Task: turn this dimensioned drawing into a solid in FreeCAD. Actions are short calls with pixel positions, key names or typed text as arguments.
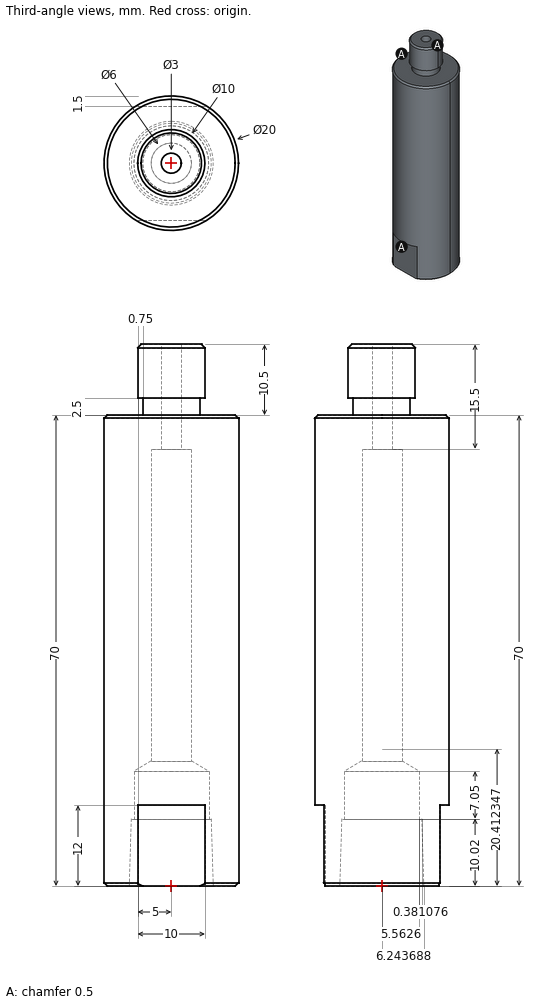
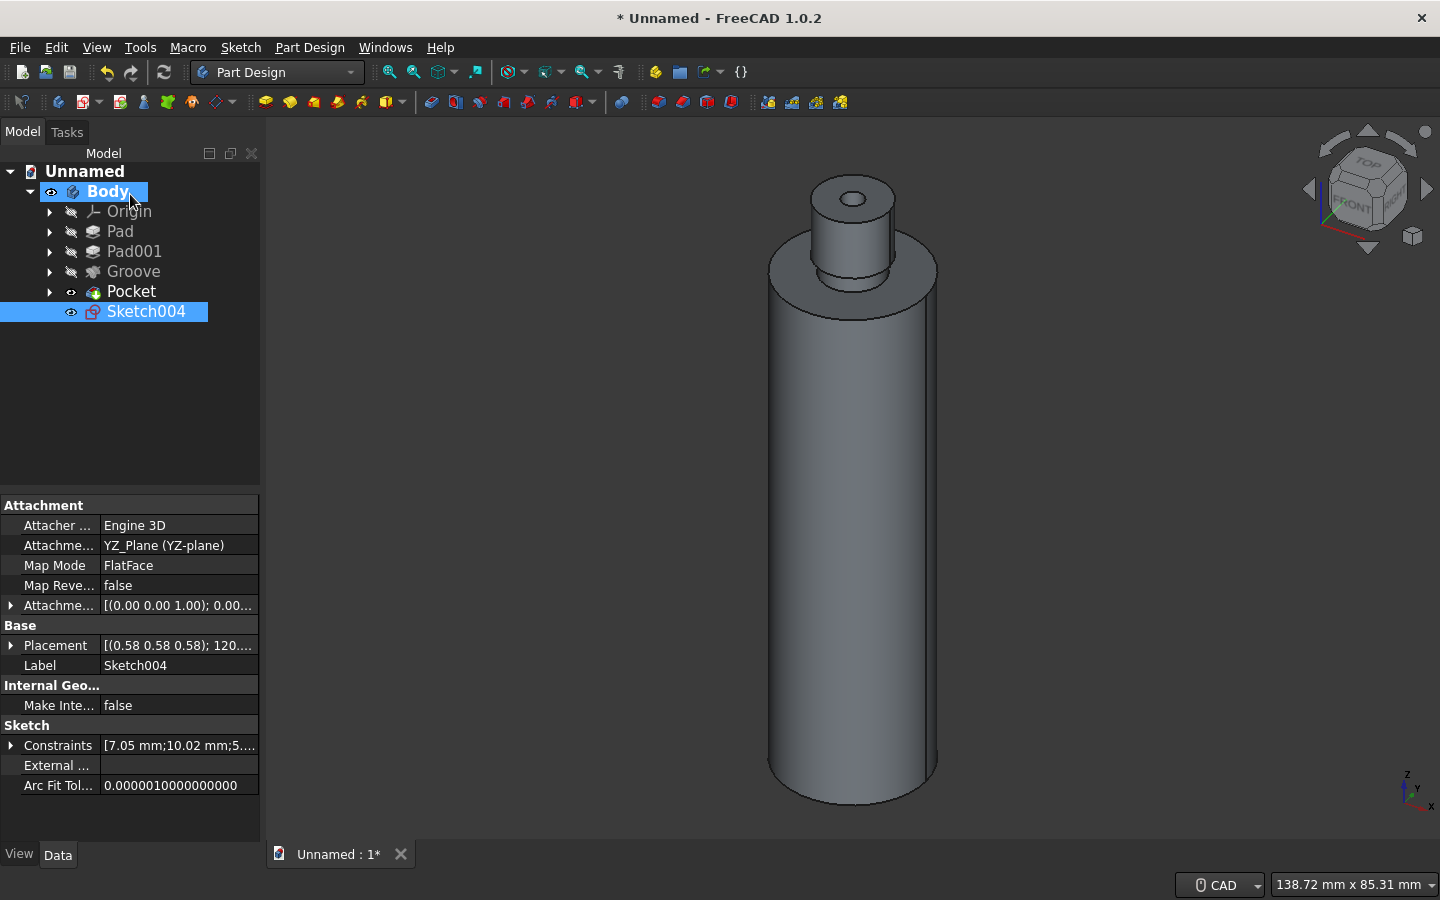
click(480, 102)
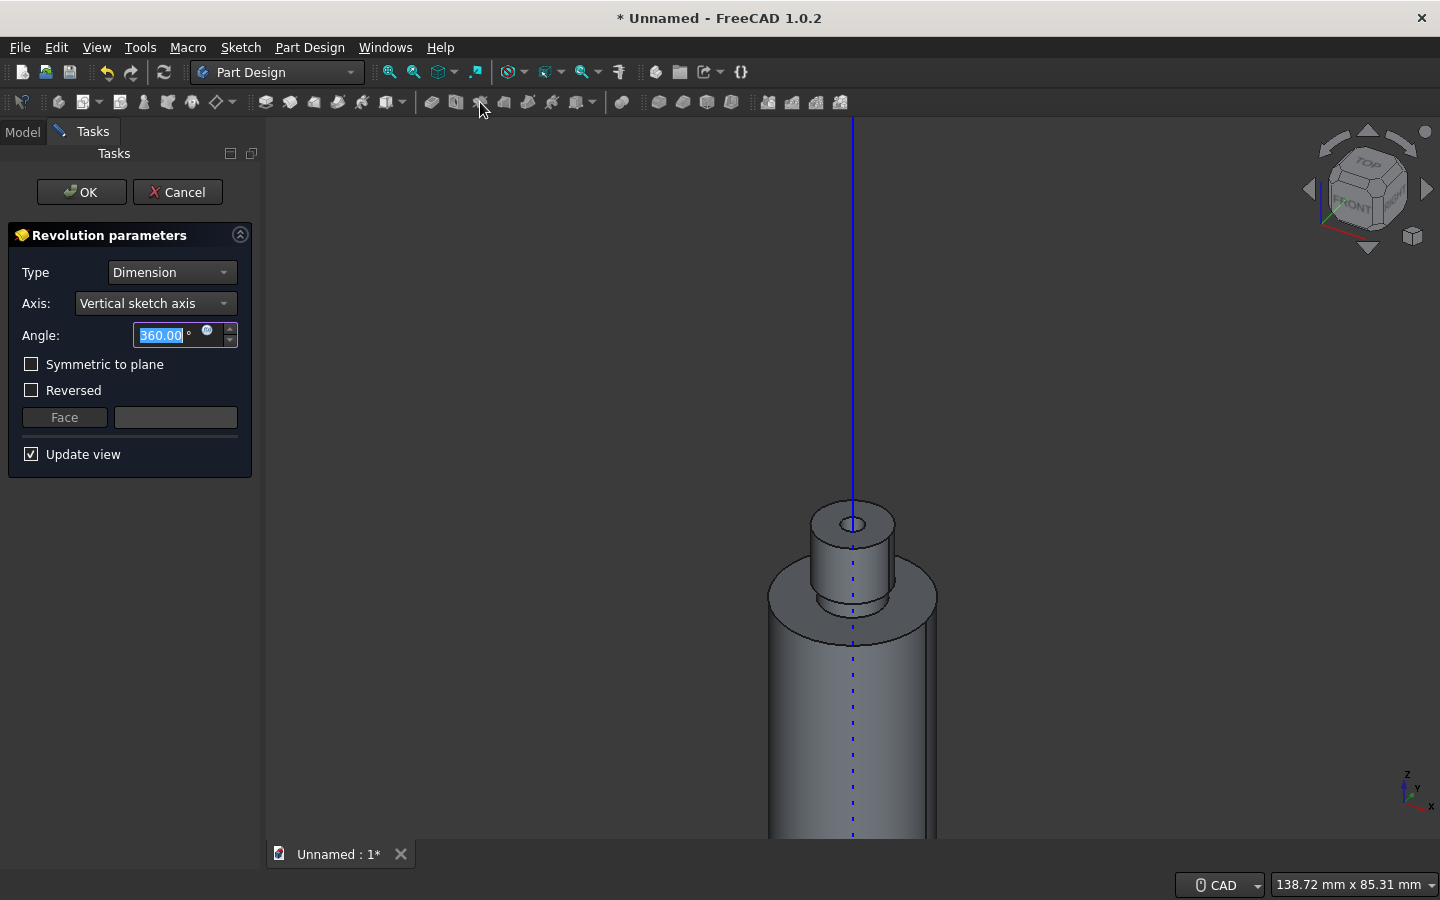
click(82, 192)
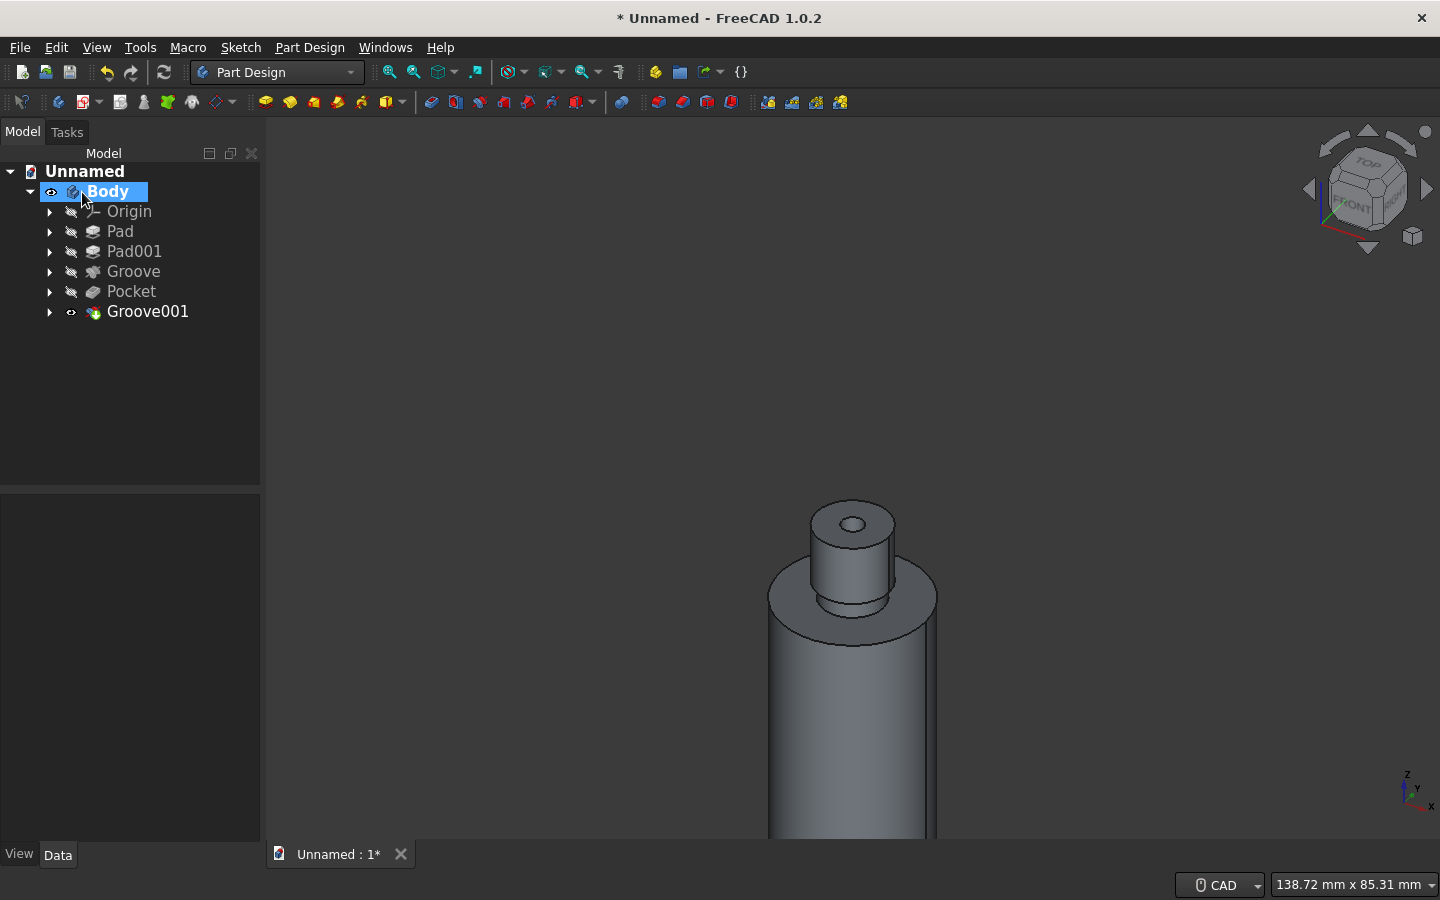
click(390, 72)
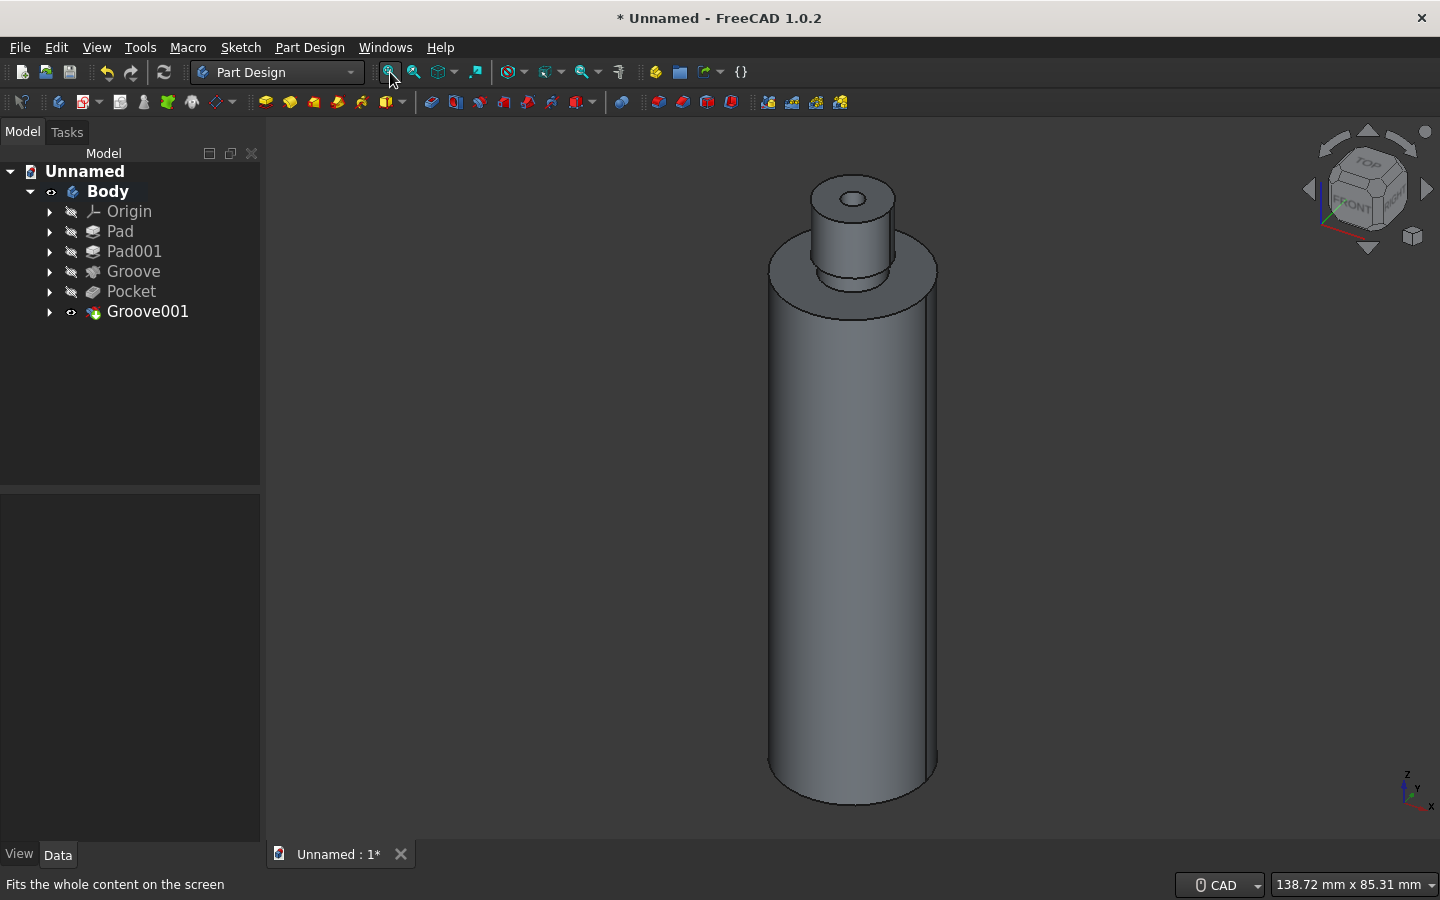
key(0)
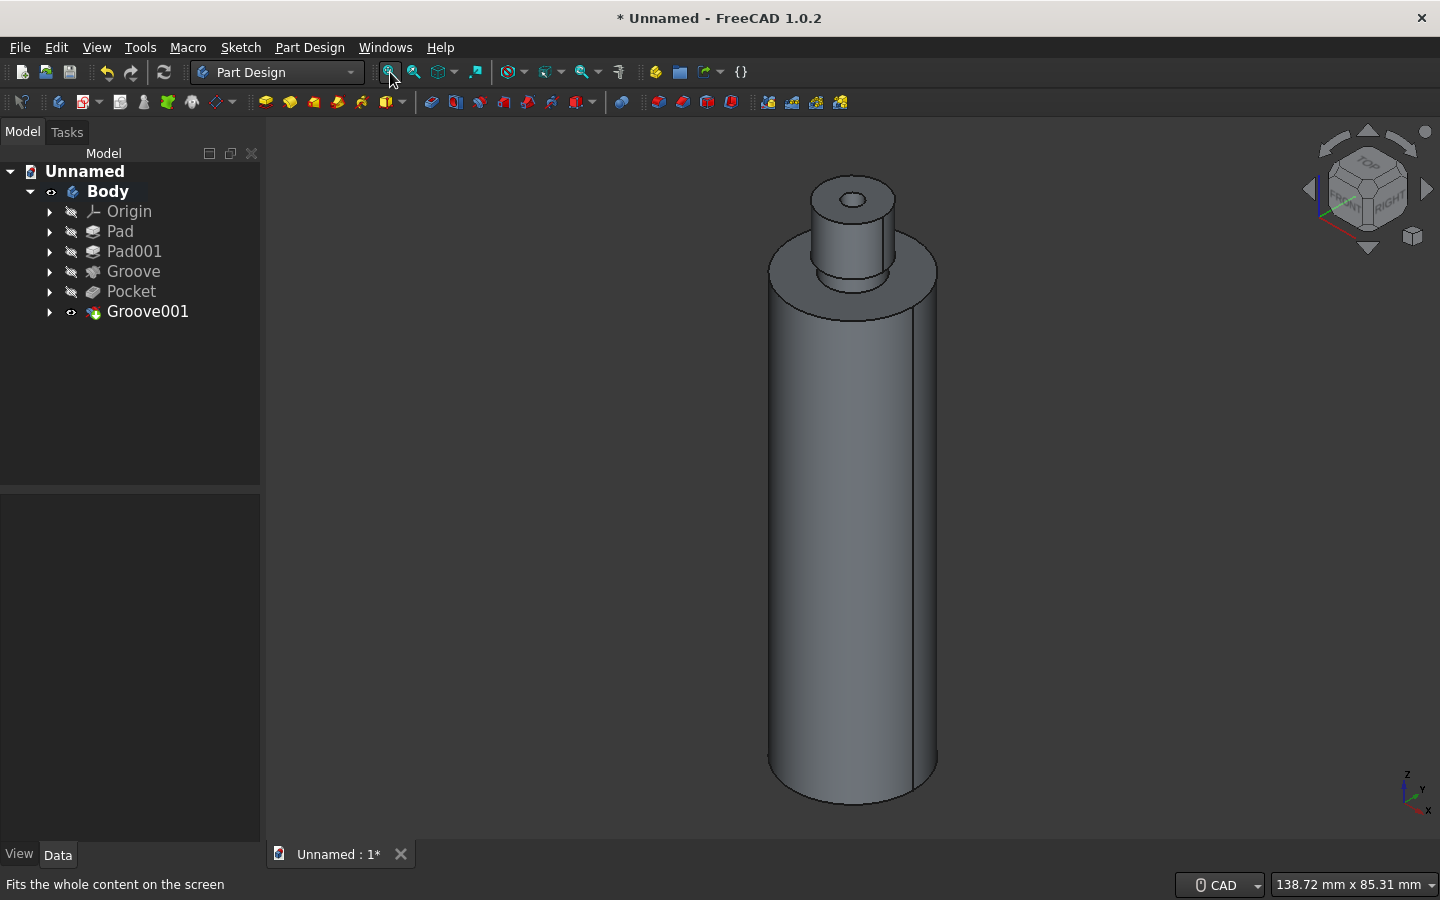
key(2)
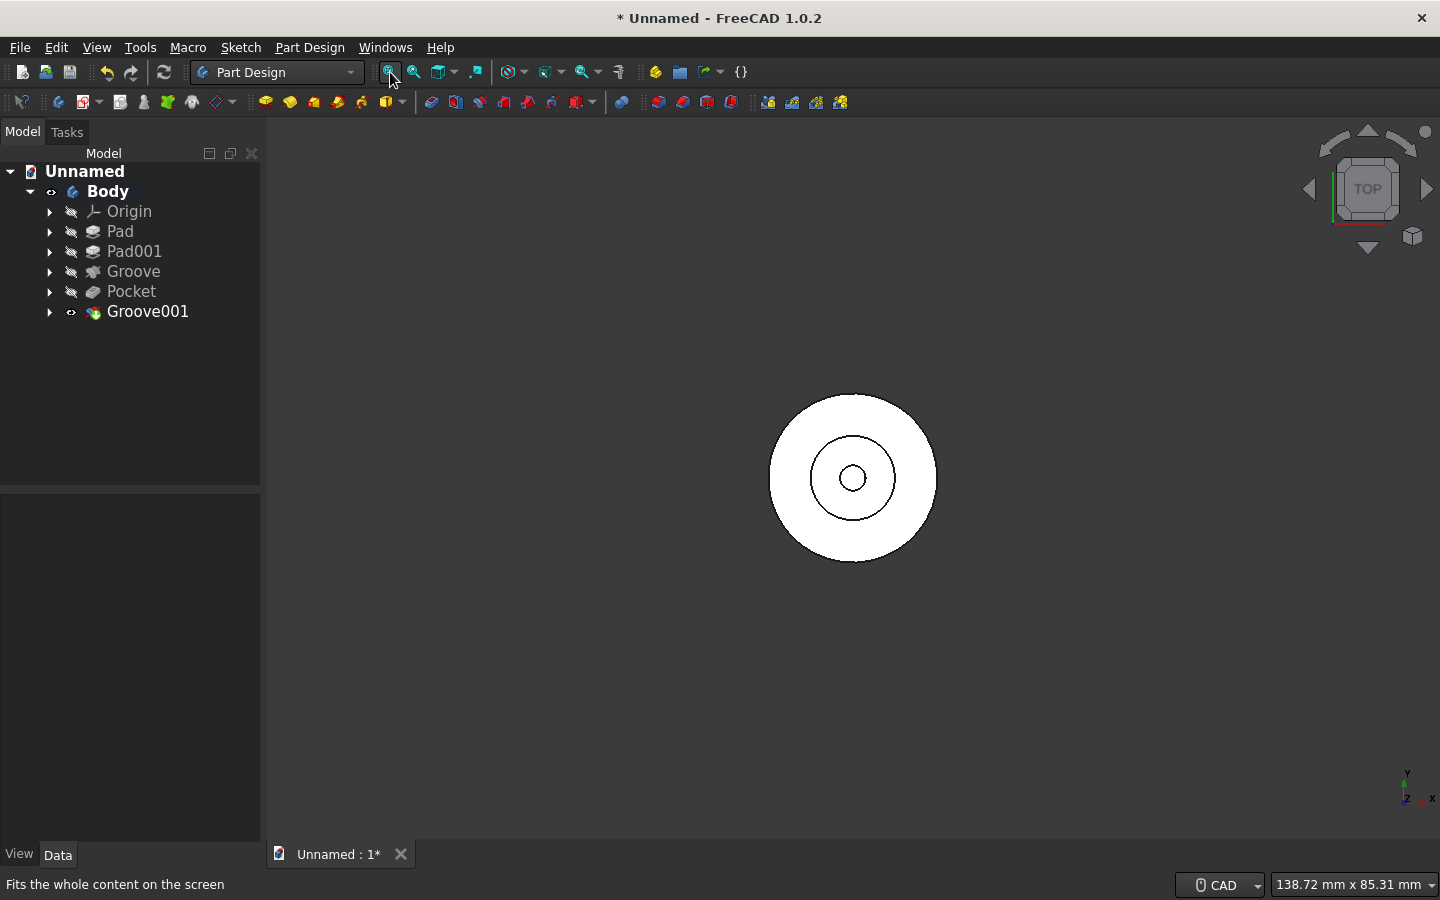
click(390, 72)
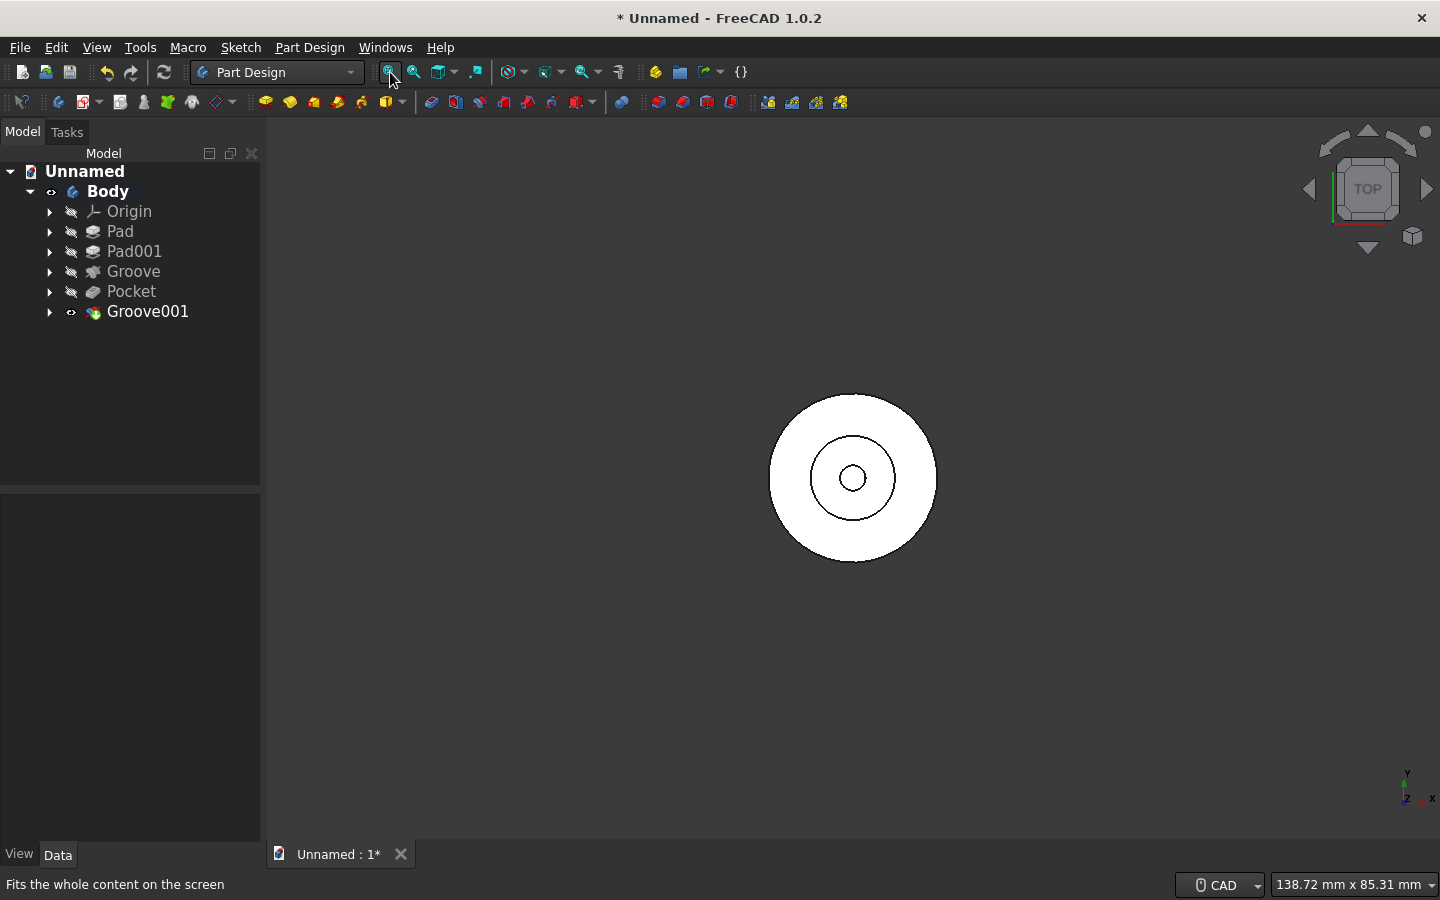
click(853, 477)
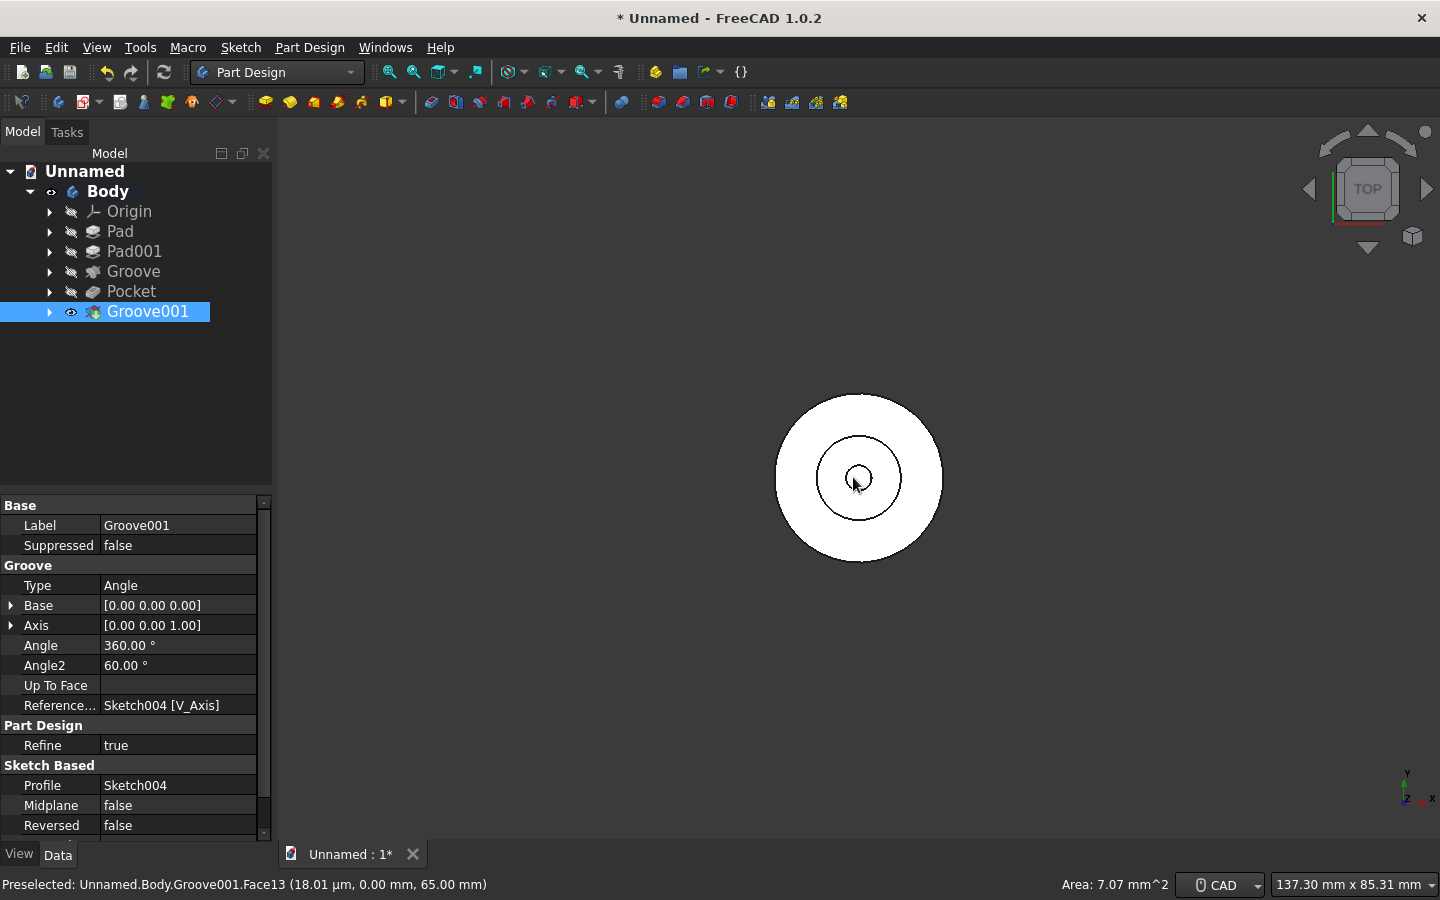
click(84, 102)